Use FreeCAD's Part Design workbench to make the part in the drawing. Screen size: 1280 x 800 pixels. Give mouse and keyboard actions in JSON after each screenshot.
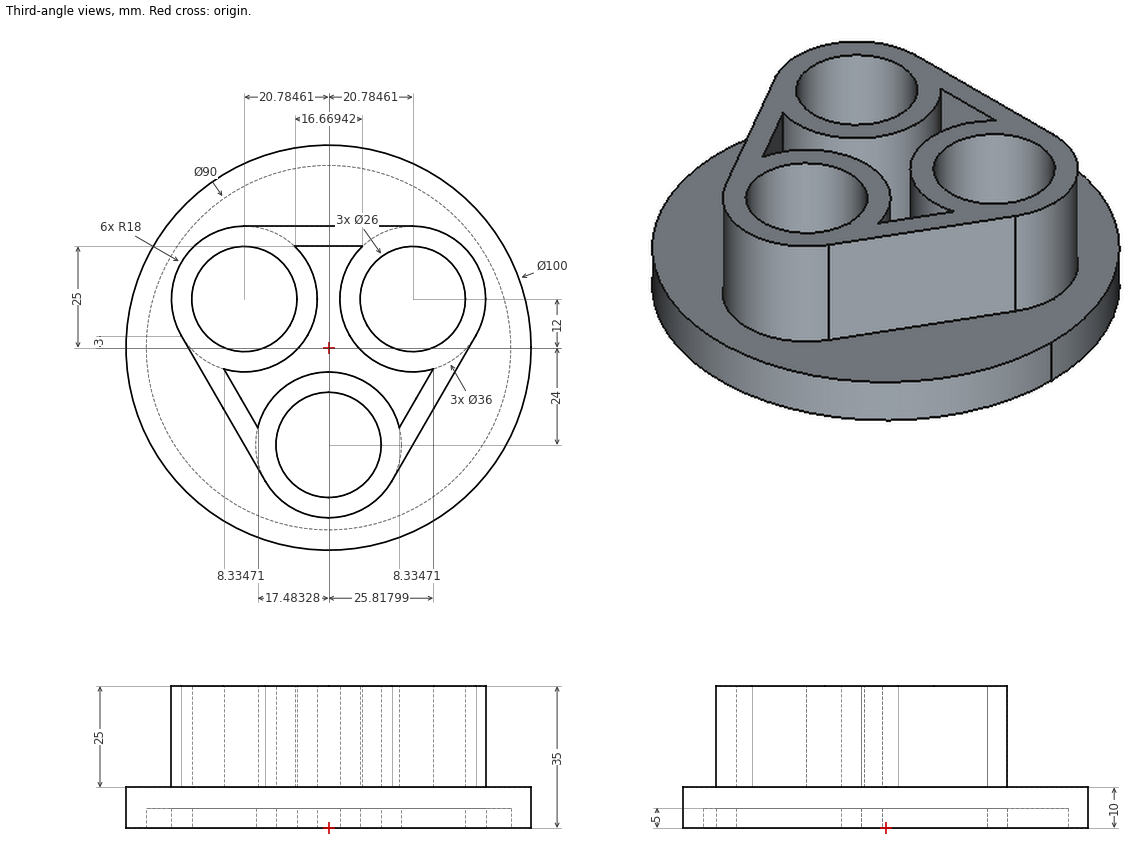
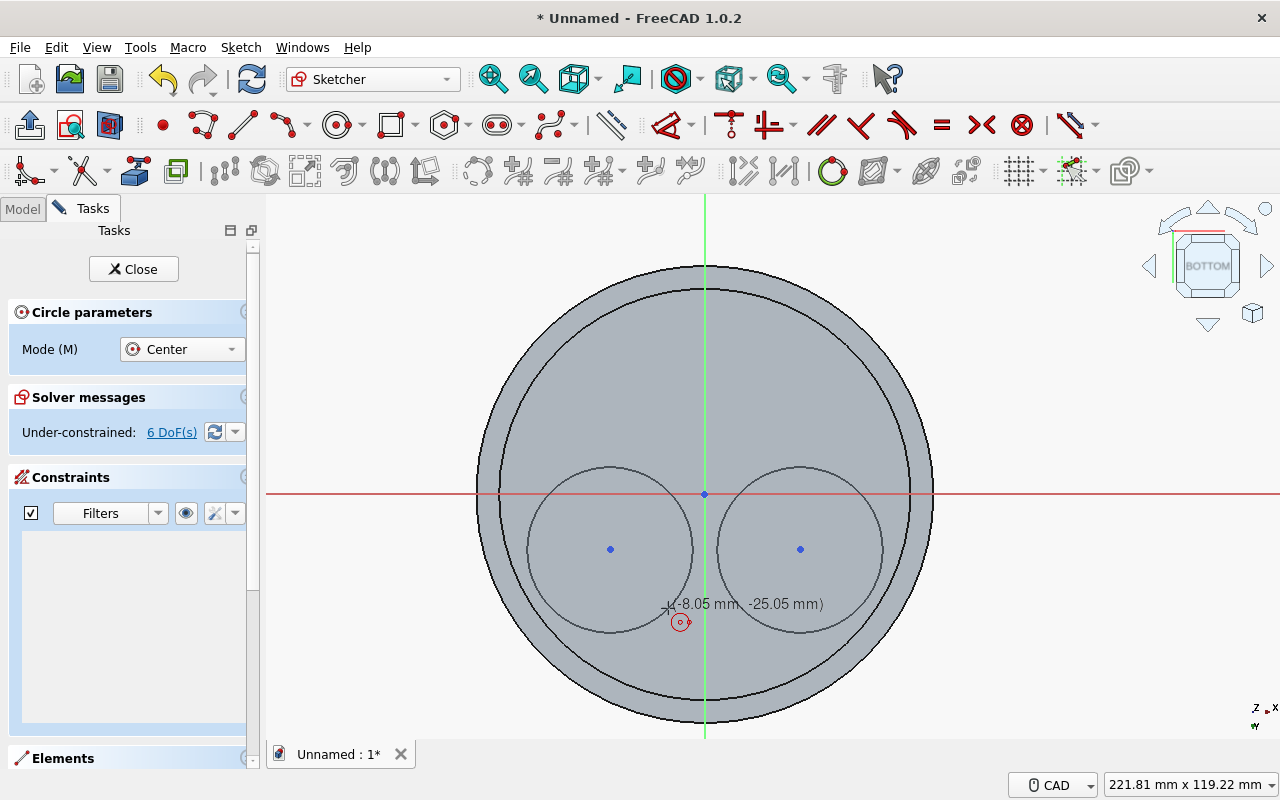
{"action": "left_click", "coordinate": [705, 385]}
{"action": "left_click", "coordinate": [763, 327]}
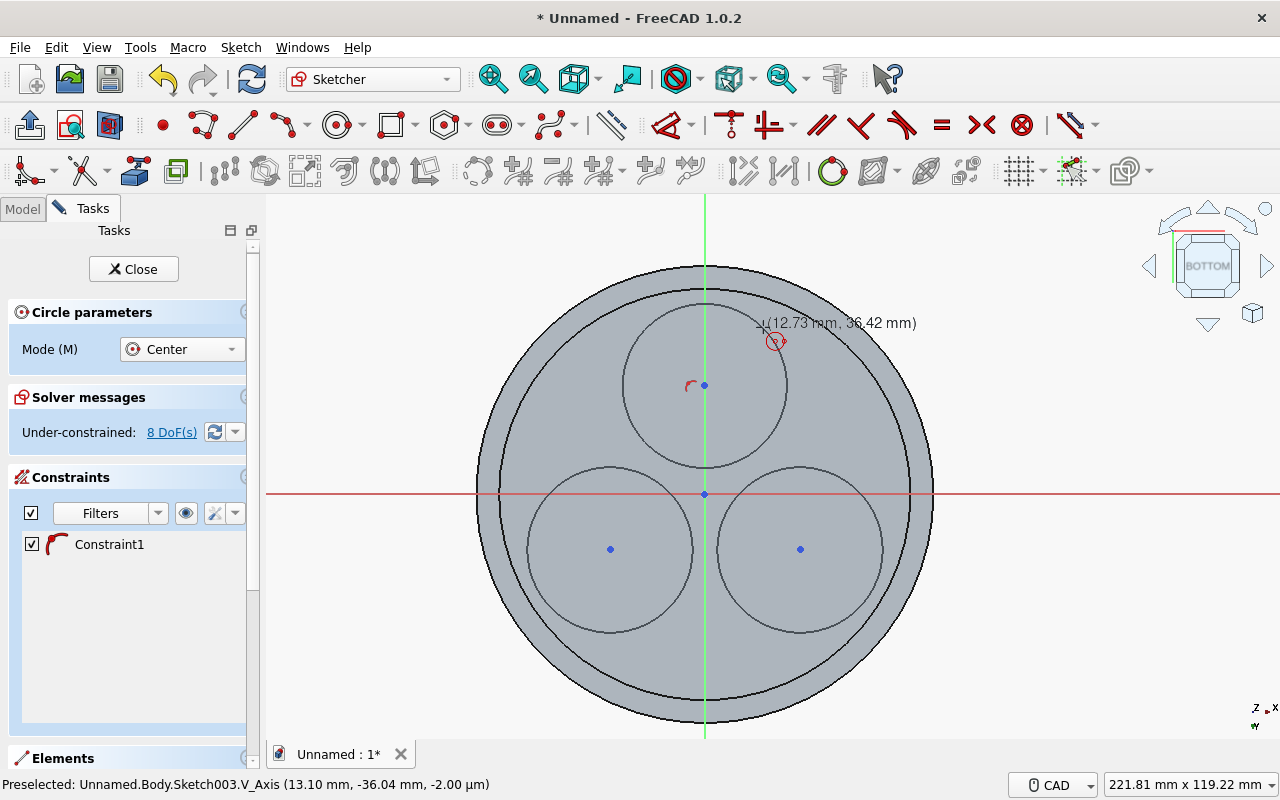
{"action": "left_click", "coordinate": [800, 550]}
{"action": "left_click", "coordinate": [842, 591]}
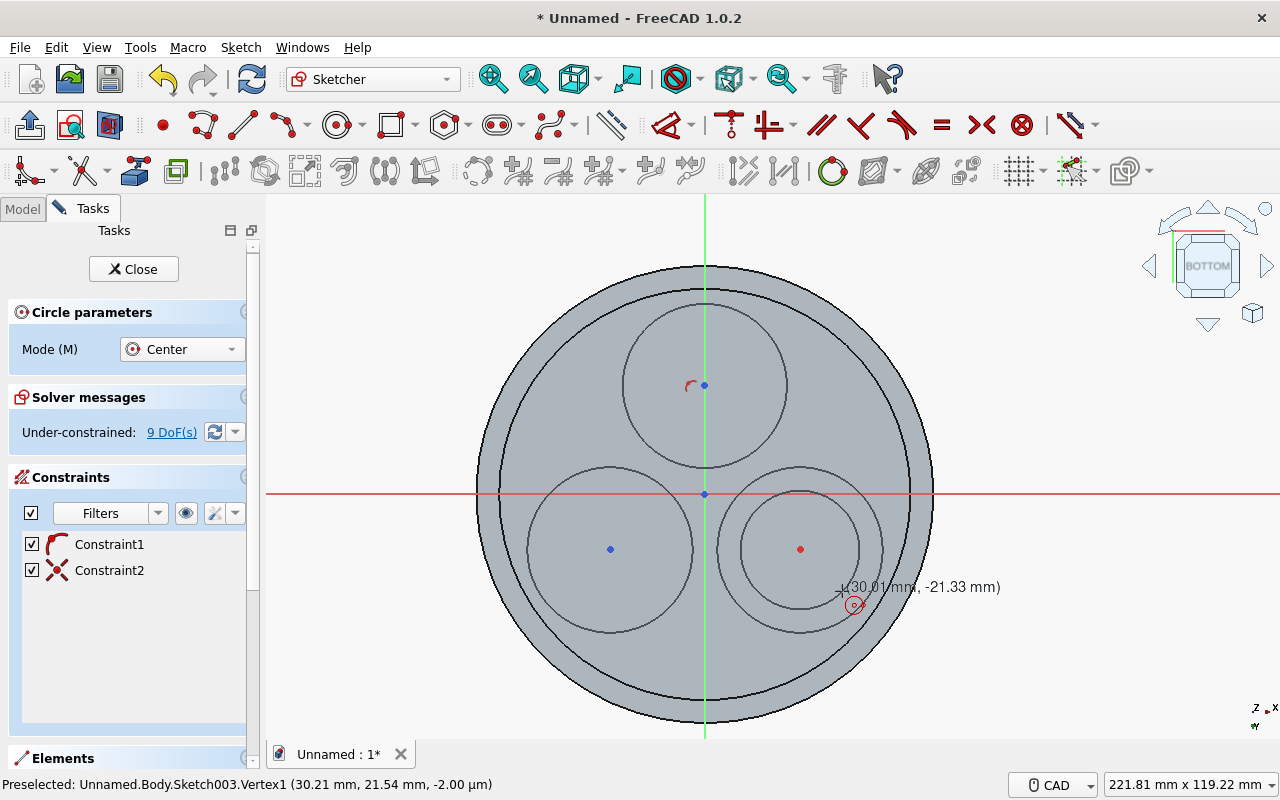
{"action": "left_click", "coordinate": [610, 550]}
{"action": "left_click", "coordinate": [652, 591]}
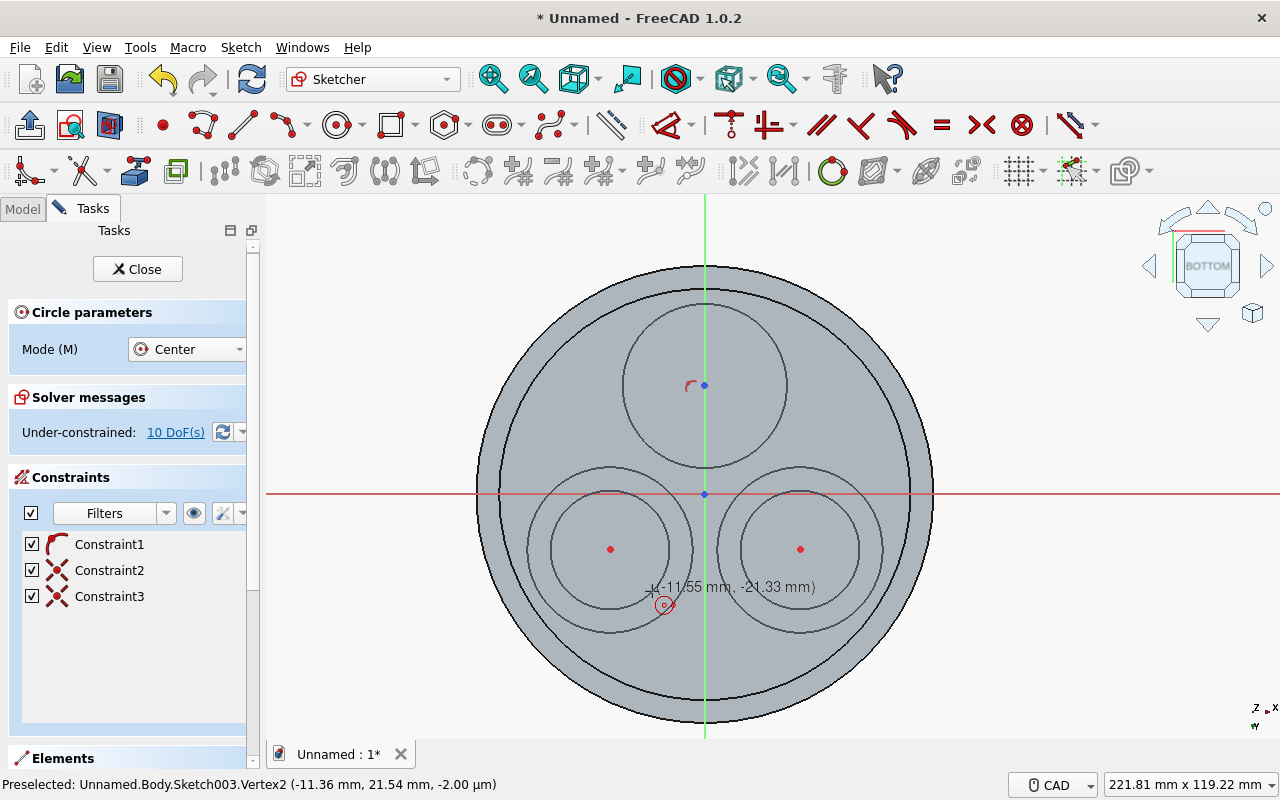
{"action": "left_click", "coordinate": [705, 386]}
{"action": "left_click", "coordinate": [747, 343]}
{"action": "key", "text": "Escape"}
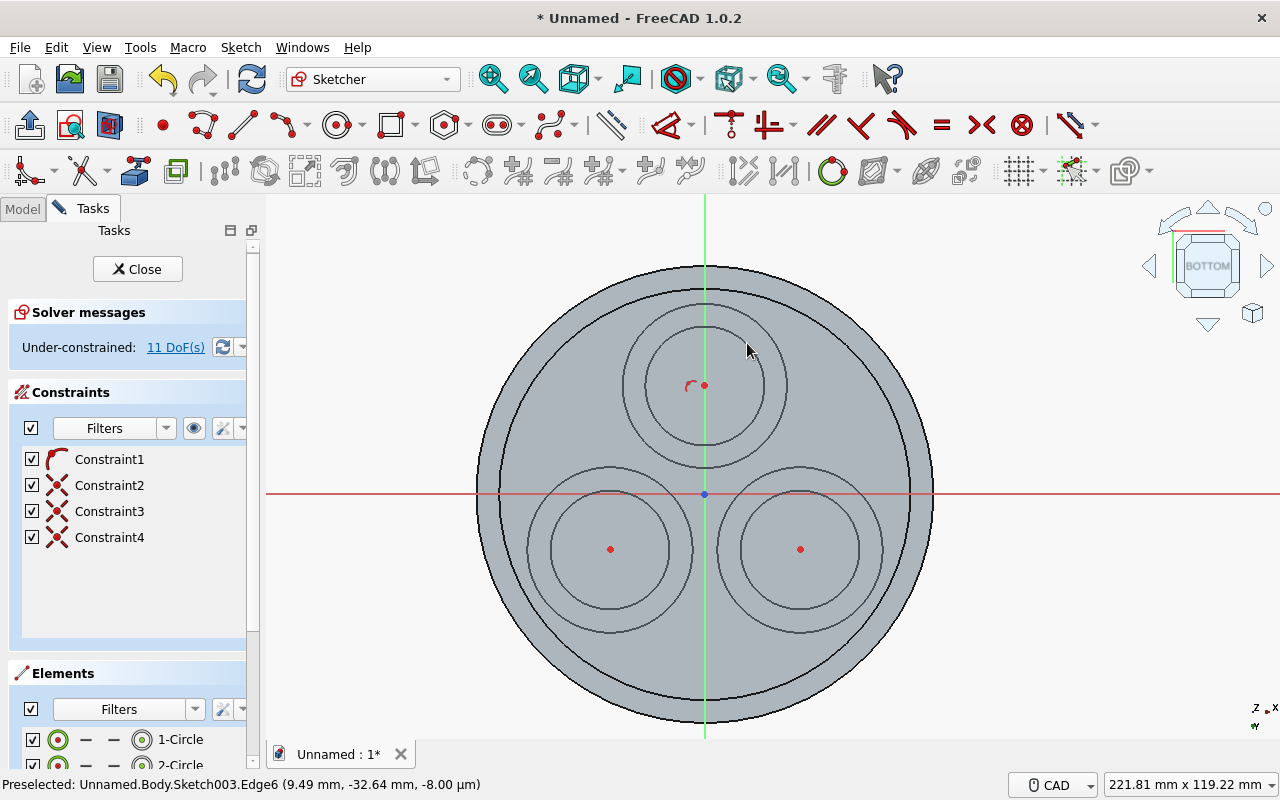
{"action": "left_click", "coordinate": [858, 491]}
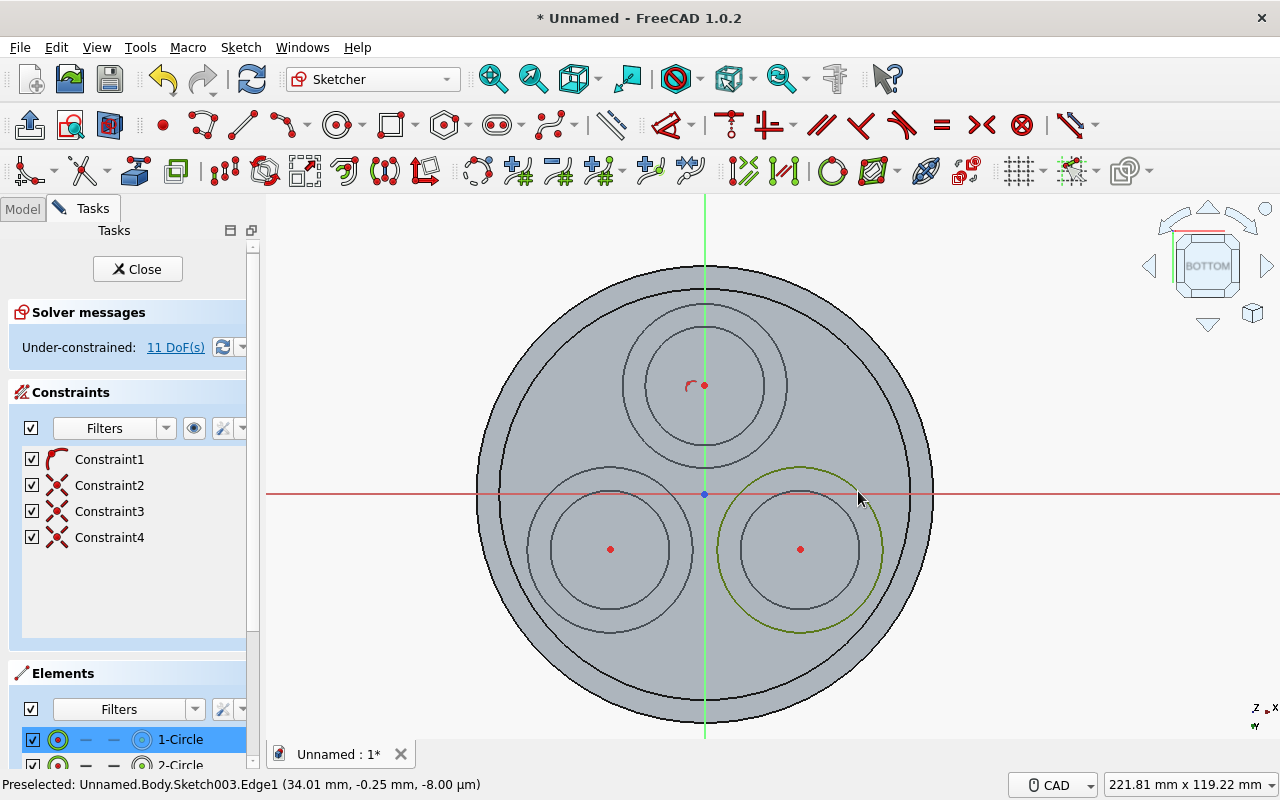
{"action": "left_click", "coordinate": [668, 491]}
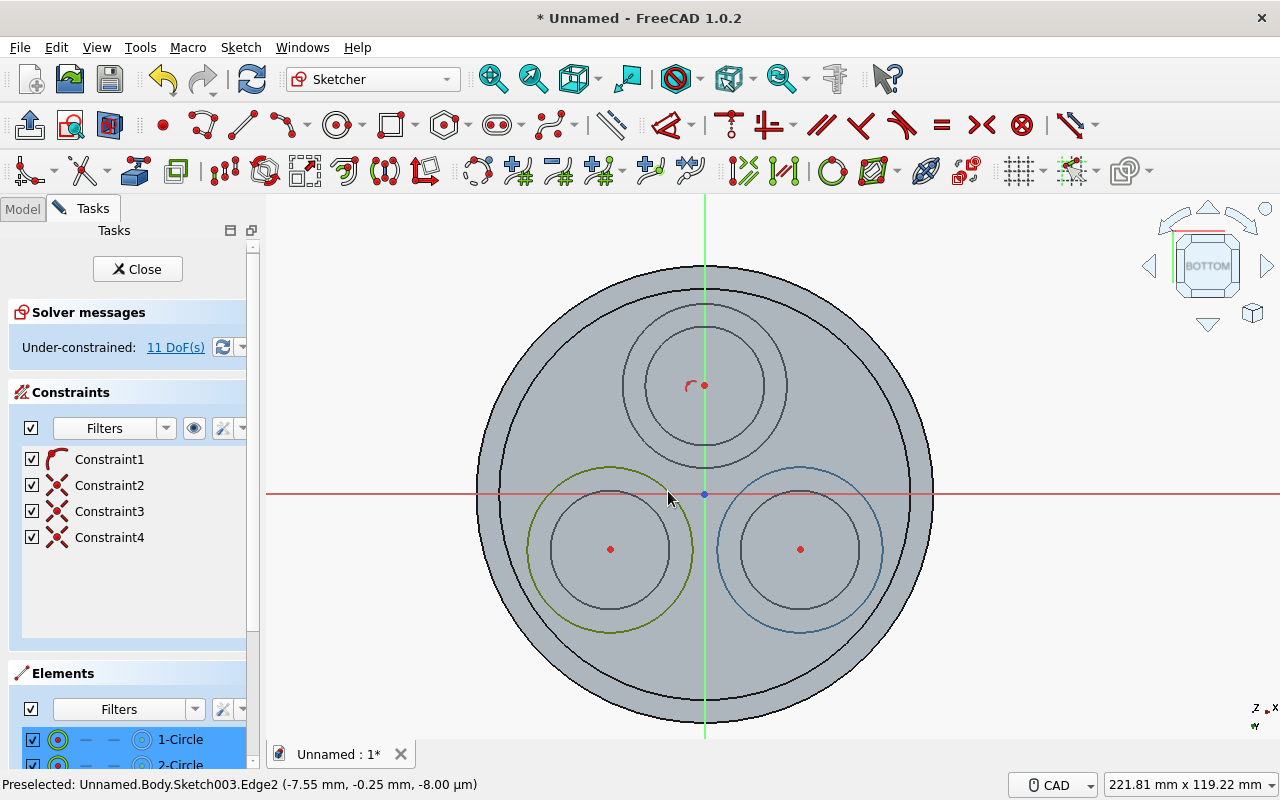
{"action": "left_click", "coordinate": [763, 328]}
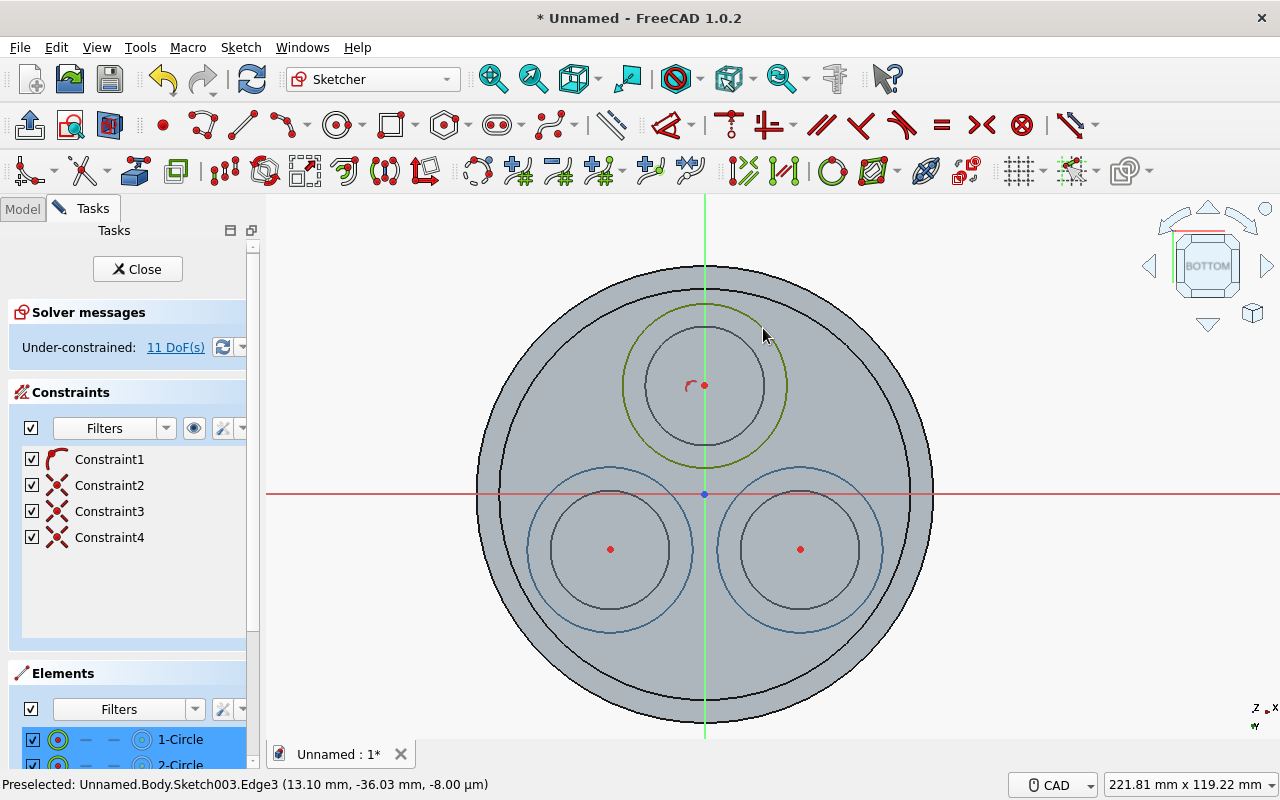
{"action": "left_click", "coordinate": [942, 126]}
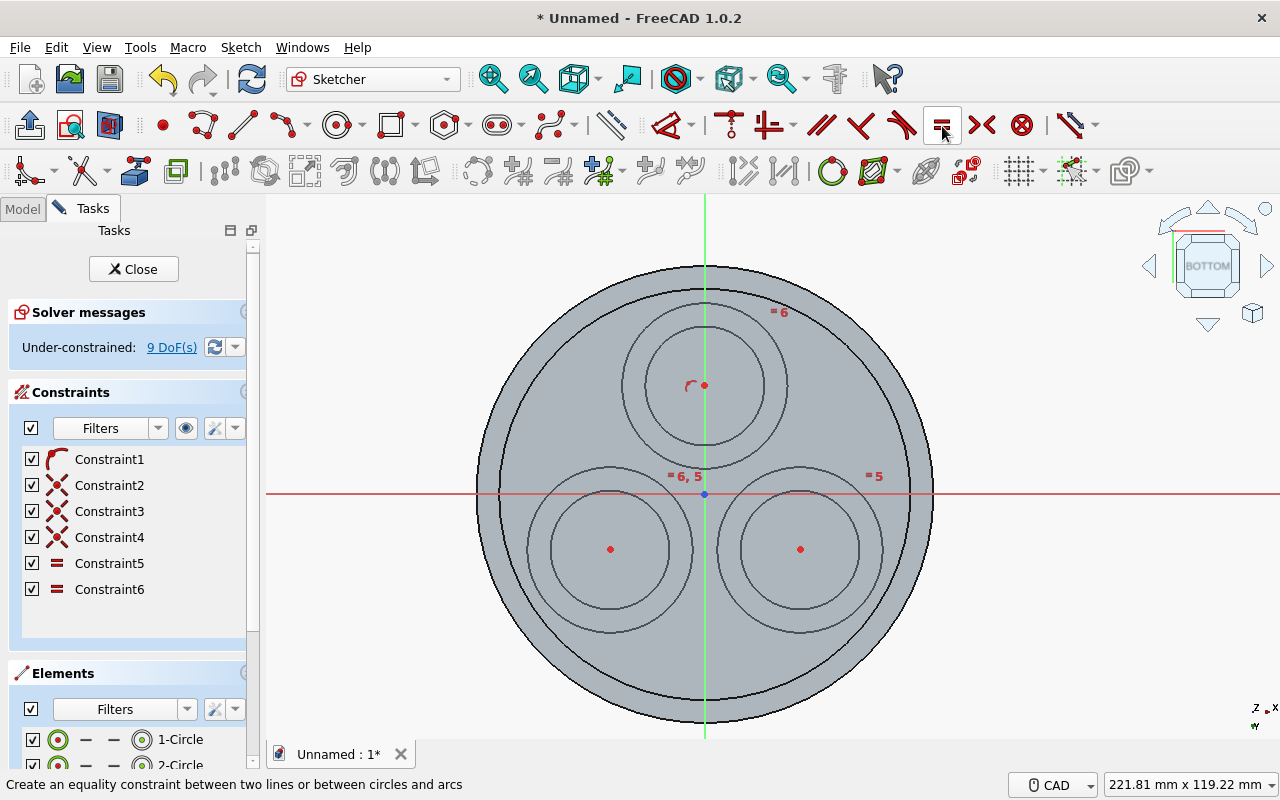
{"action": "left_click", "coordinate": [842, 508]}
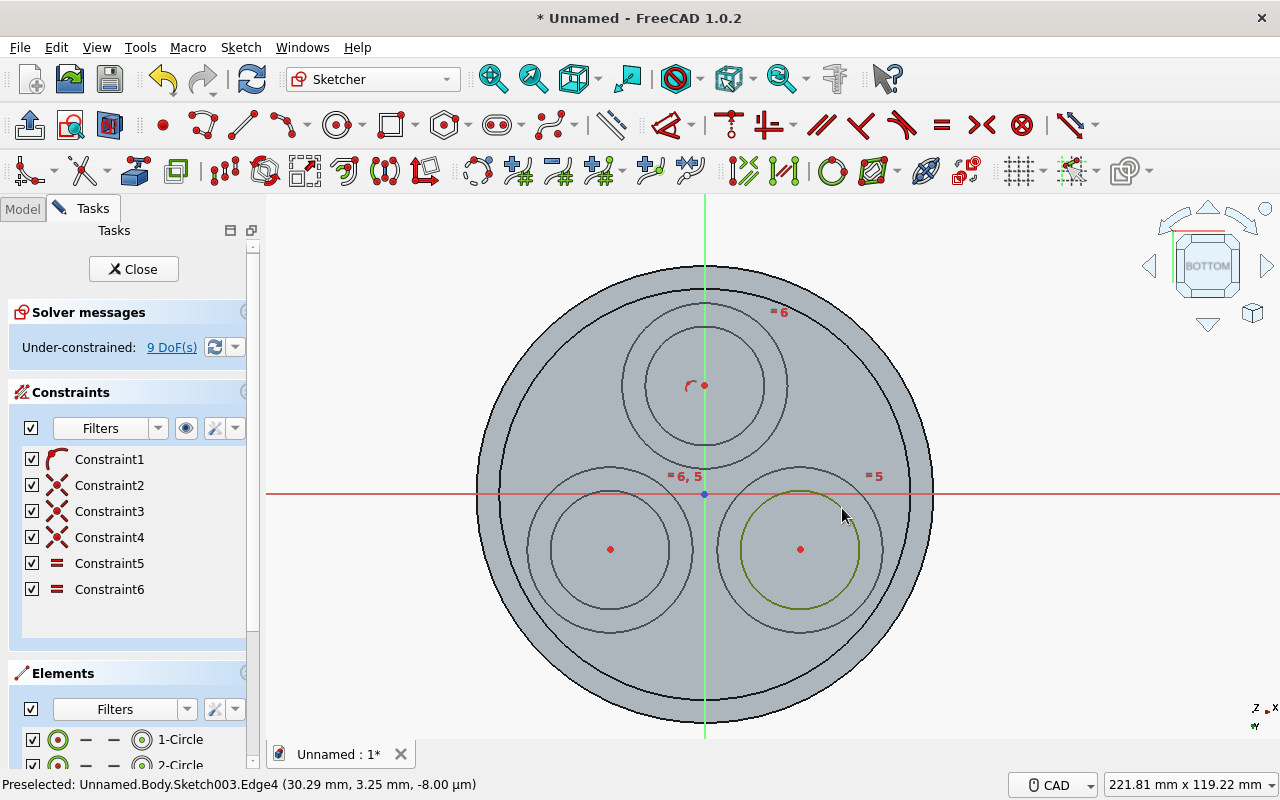
{"action": "left_click", "coordinate": [652, 508]}